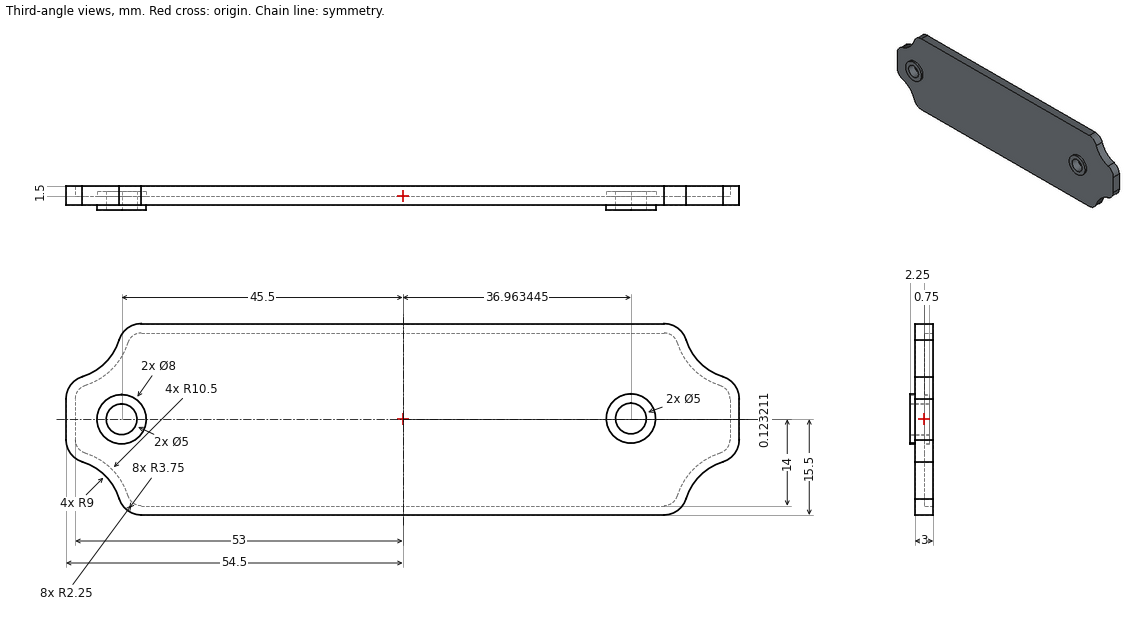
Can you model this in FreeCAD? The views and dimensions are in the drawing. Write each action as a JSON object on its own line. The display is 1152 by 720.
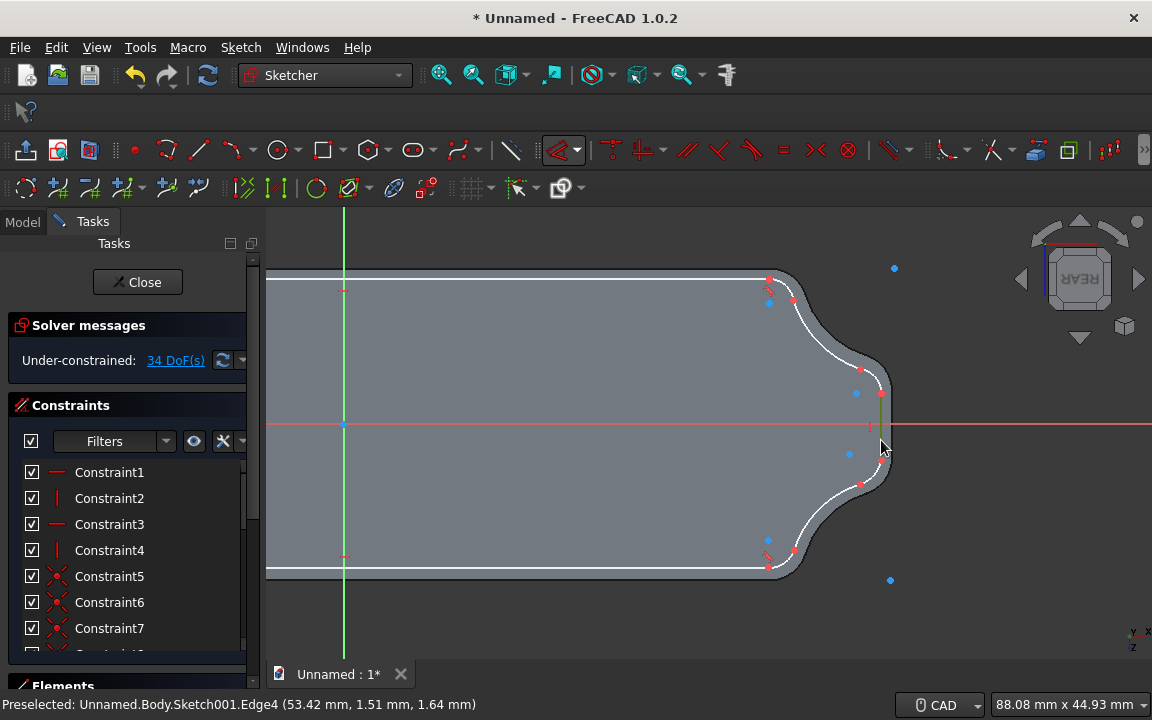
{"action": "scroll", "coordinate": [869, 480], "scroll_direction": "up", "scroll_amount": 2}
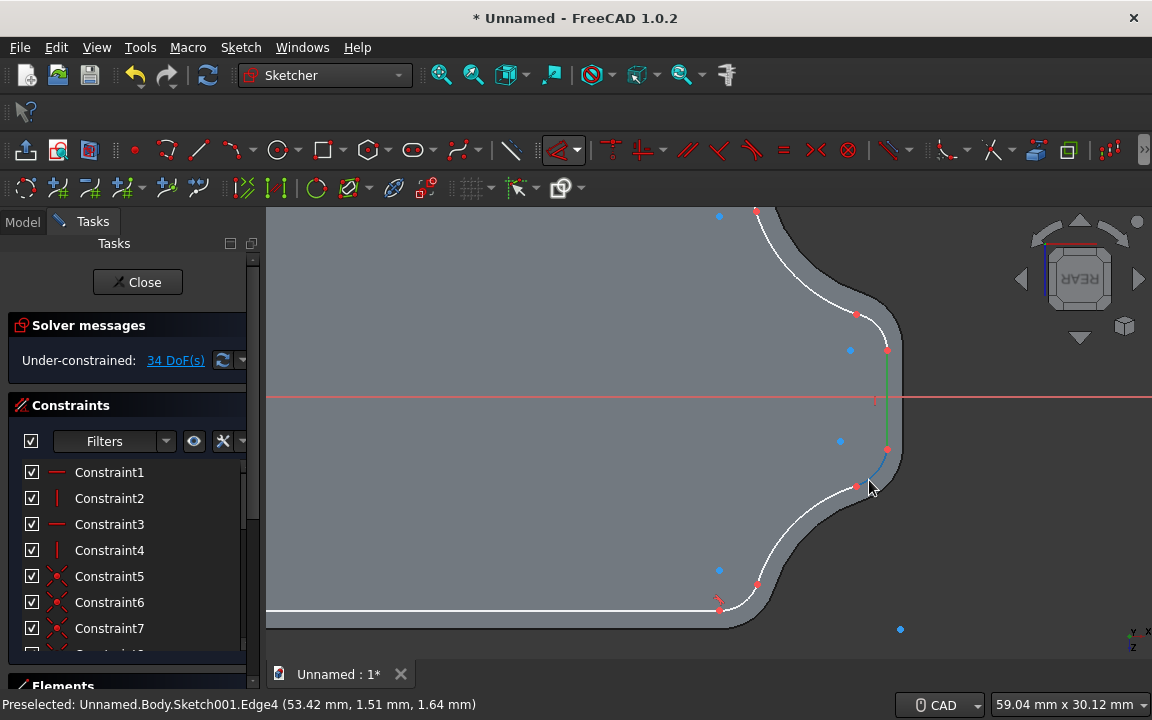
{"action": "left_click", "coordinate": [869, 479]}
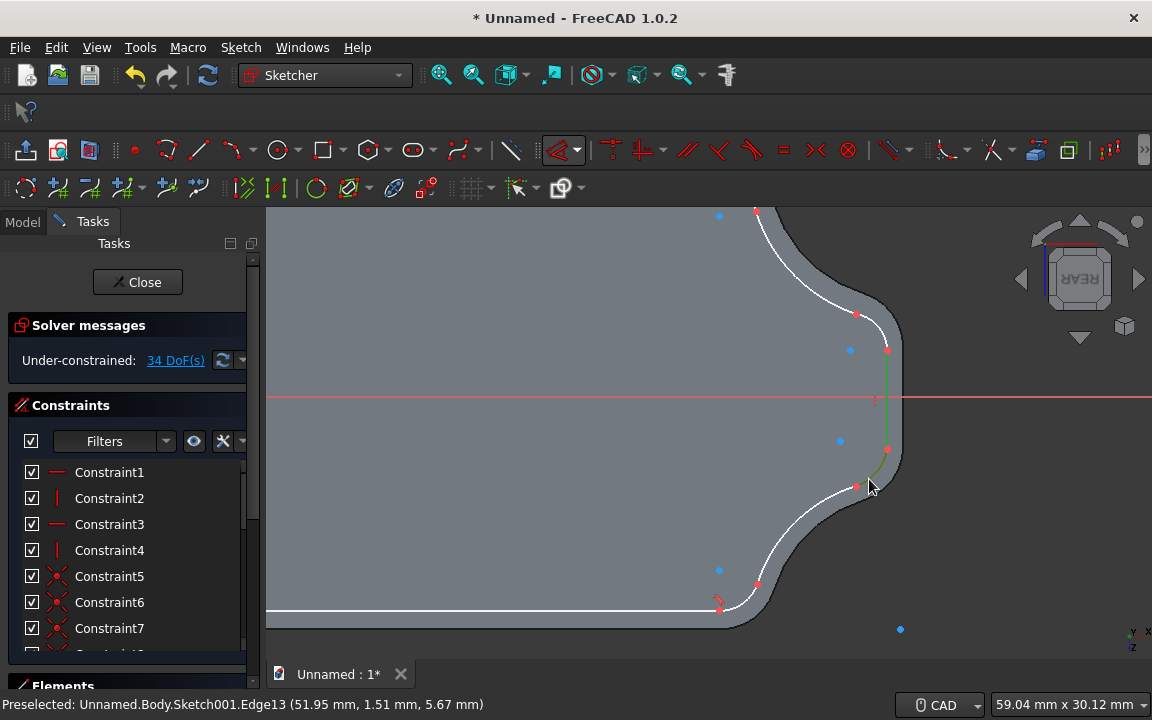
{"action": "left_click", "coordinate": [752, 150]}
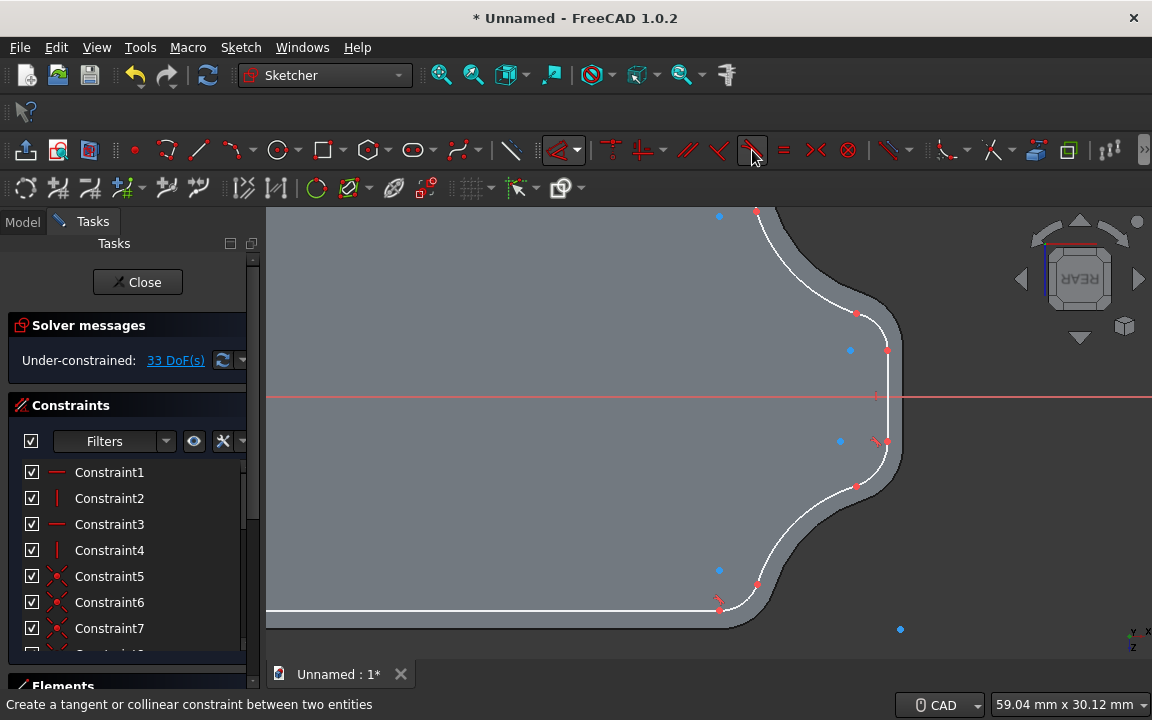
{"action": "left_click", "coordinate": [888, 414]}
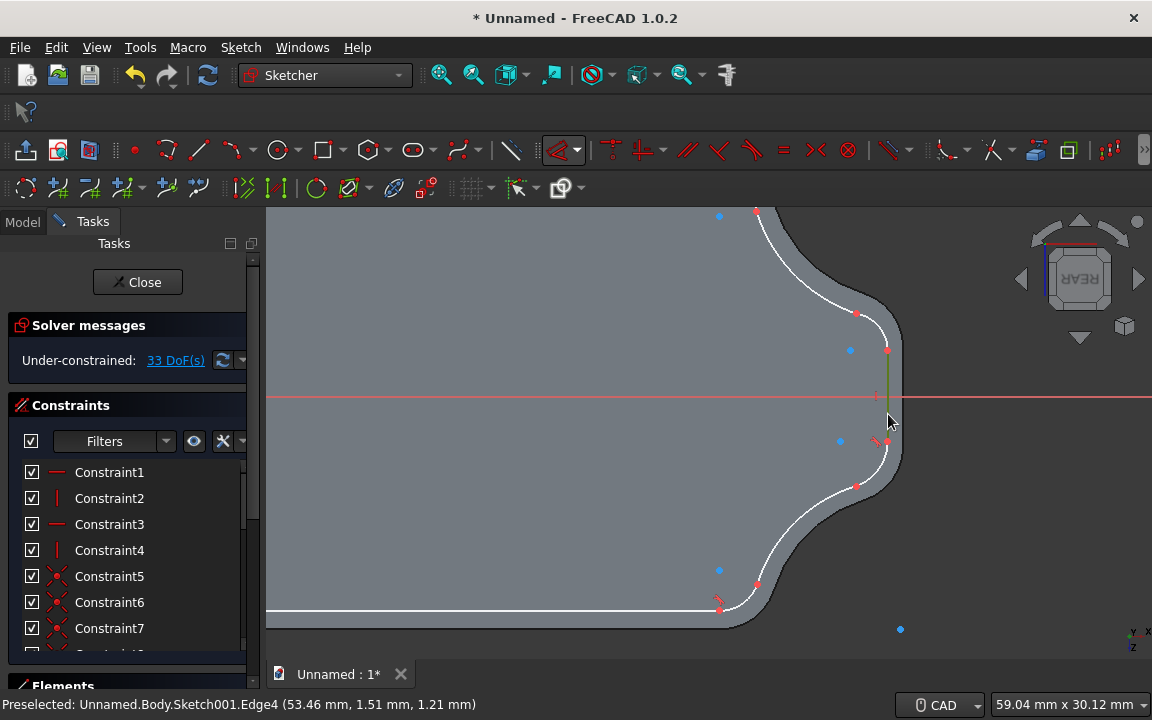
{"action": "left_click", "coordinate": [884, 335]}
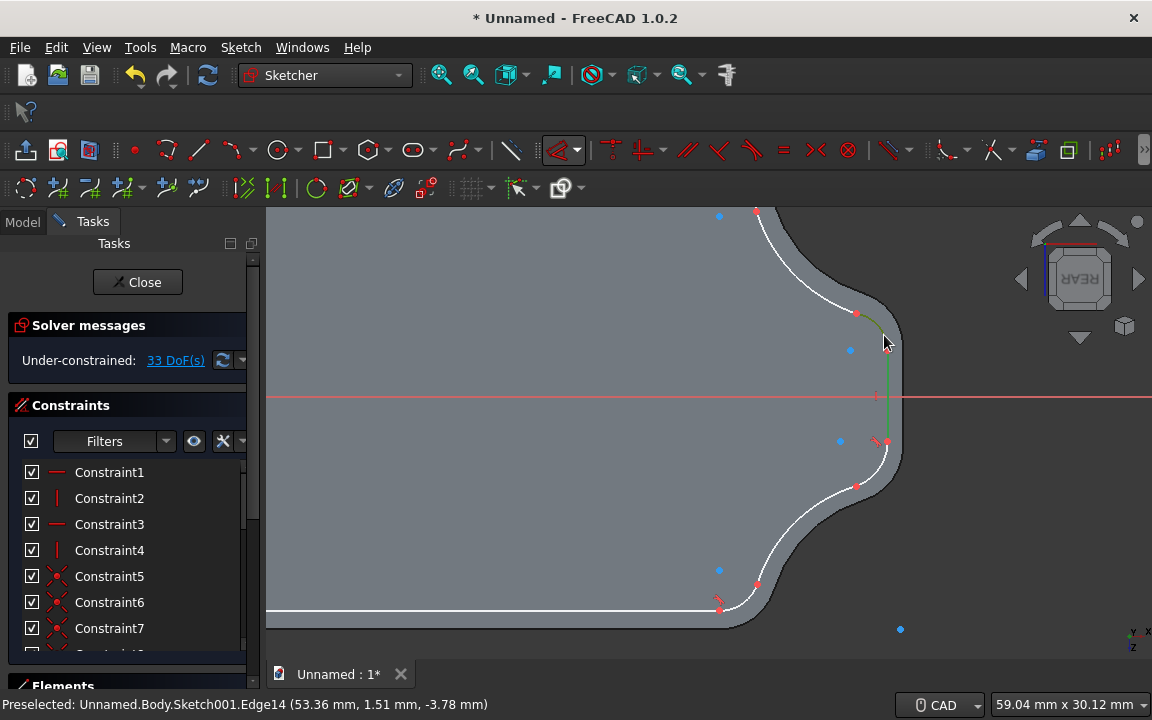
{"action": "left_click", "coordinate": [752, 150]}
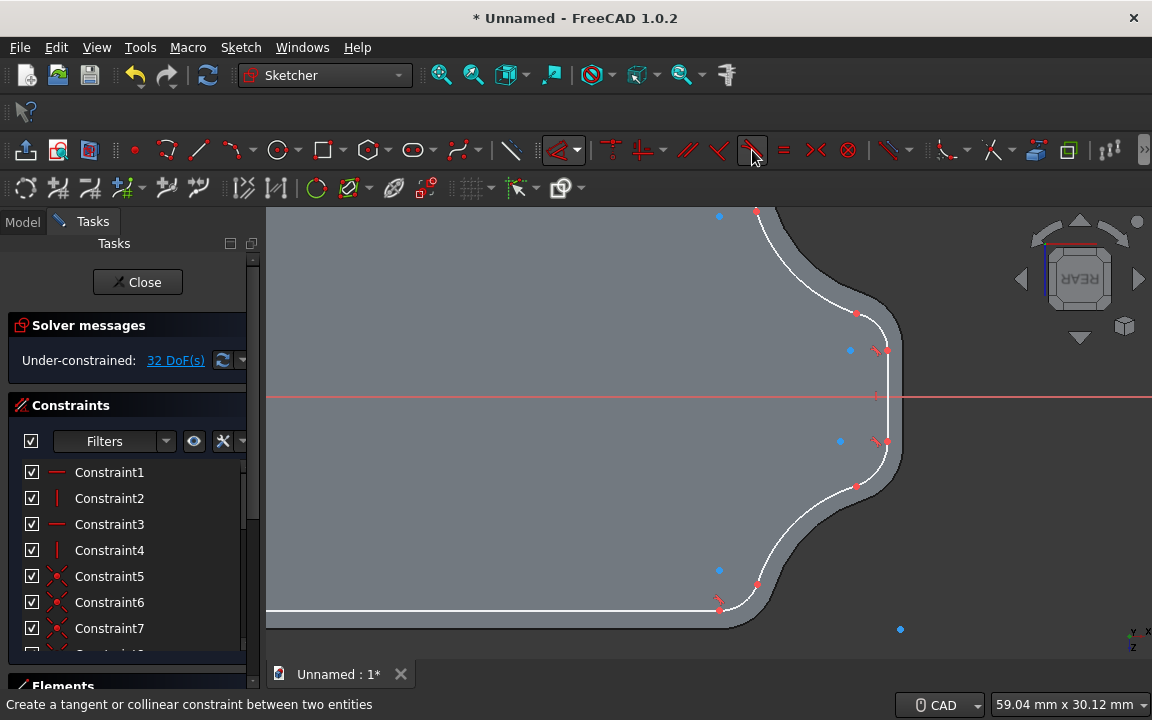
{"action": "scroll", "coordinate": [880, 449], "scroll_direction": "down", "scroll_amount": 6}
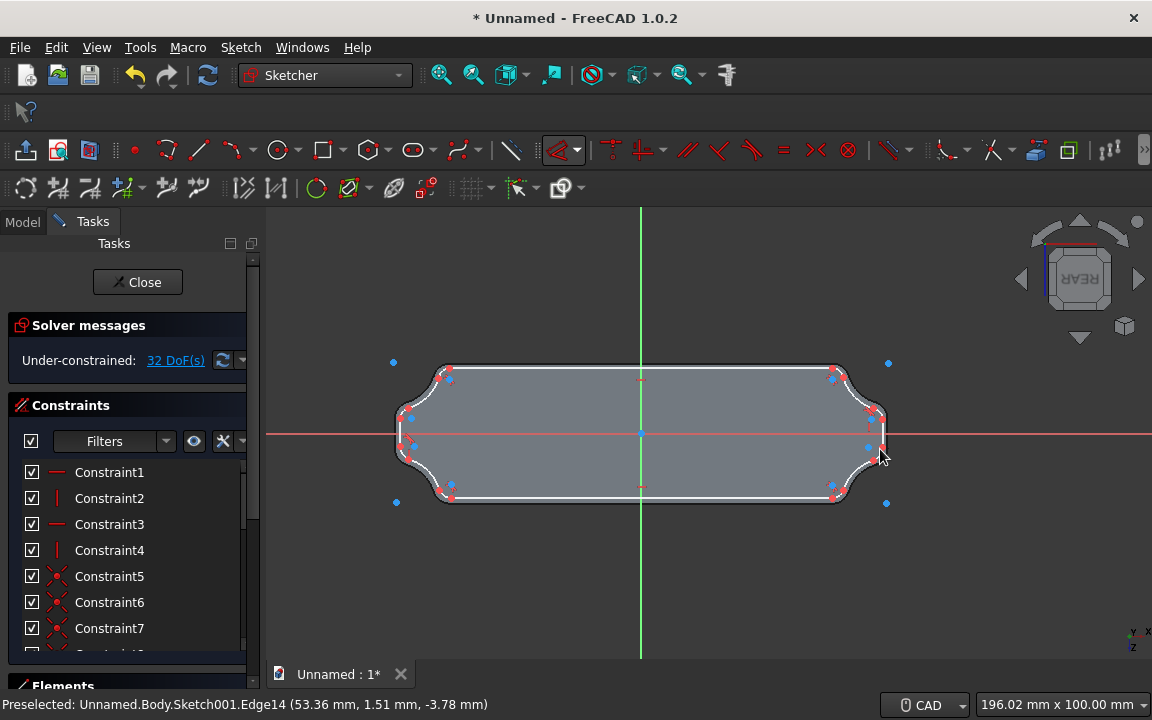
{"action": "scroll", "coordinate": [445, 369], "scroll_direction": "up", "scroll_amount": 6}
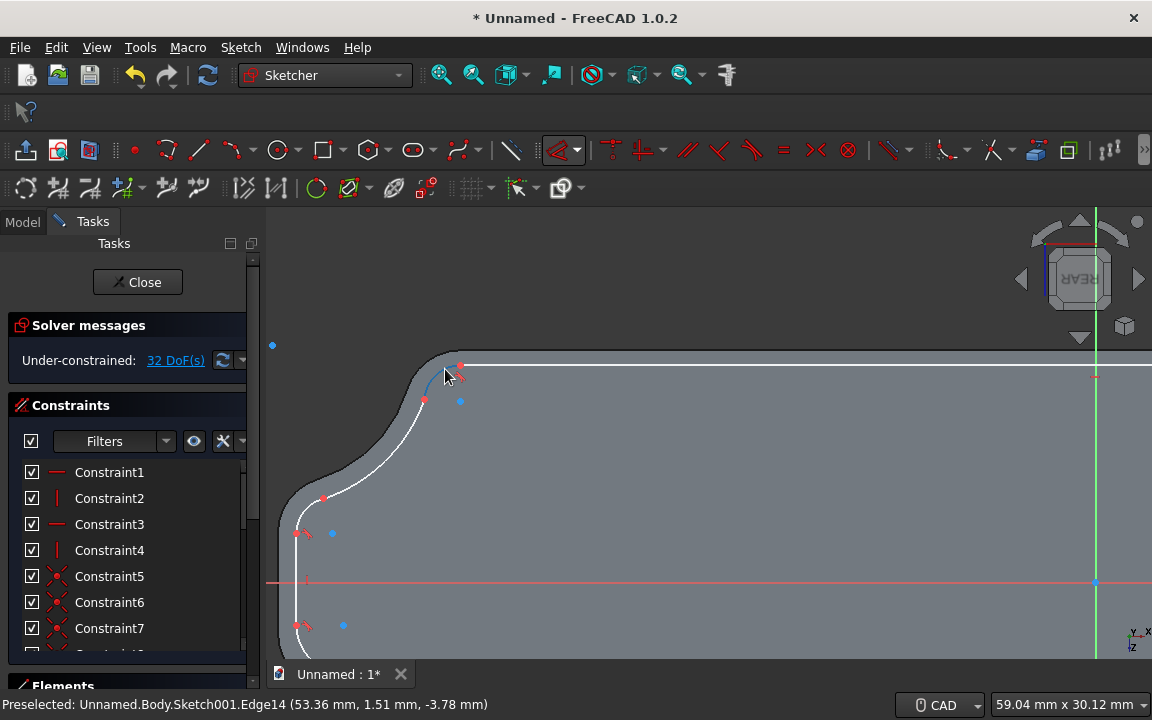
{"action": "left_click", "coordinate": [445, 369]}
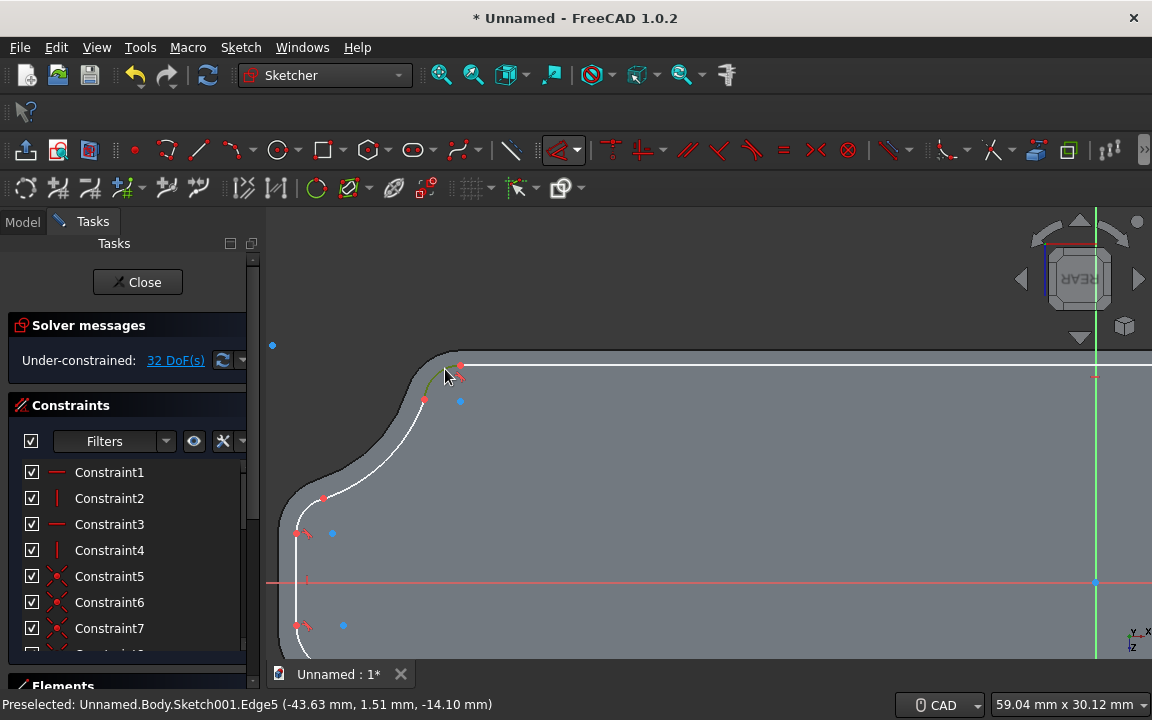
{"action": "left_click", "coordinate": [363, 479]}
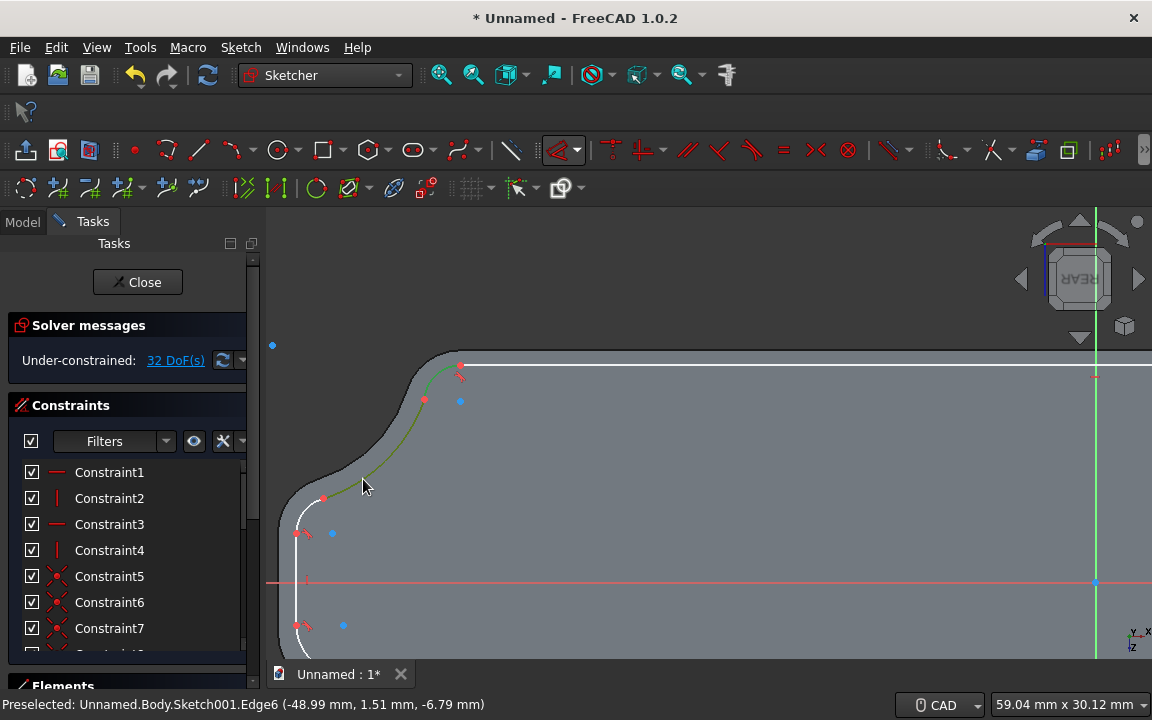
{"action": "left_click", "coordinate": [752, 150]}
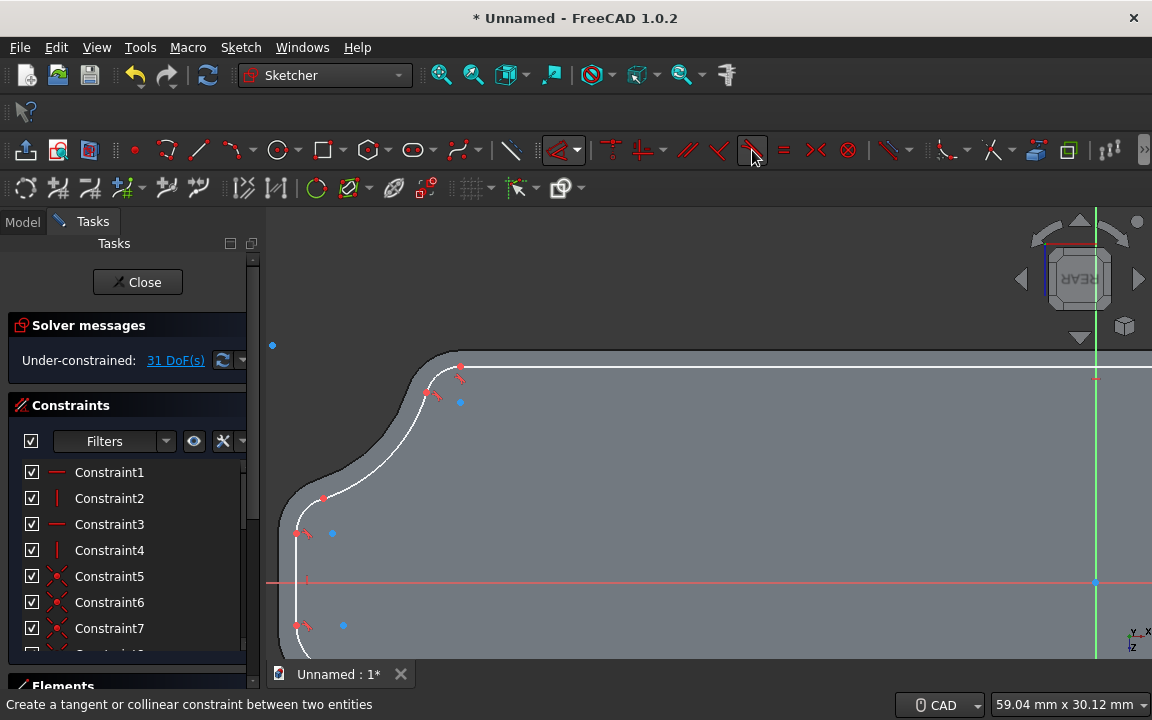
{"action": "left_click", "coordinate": [365, 478]}